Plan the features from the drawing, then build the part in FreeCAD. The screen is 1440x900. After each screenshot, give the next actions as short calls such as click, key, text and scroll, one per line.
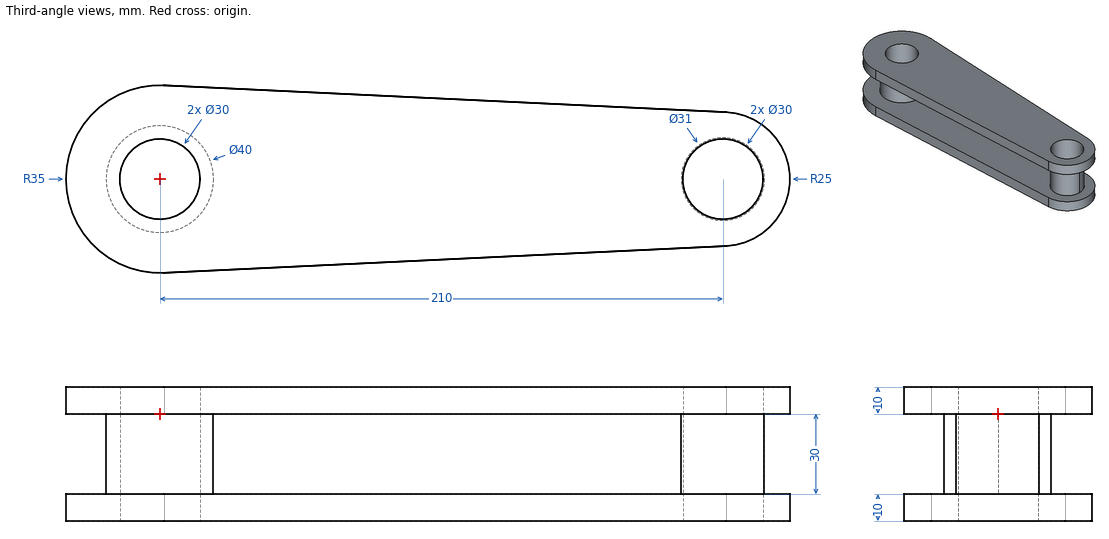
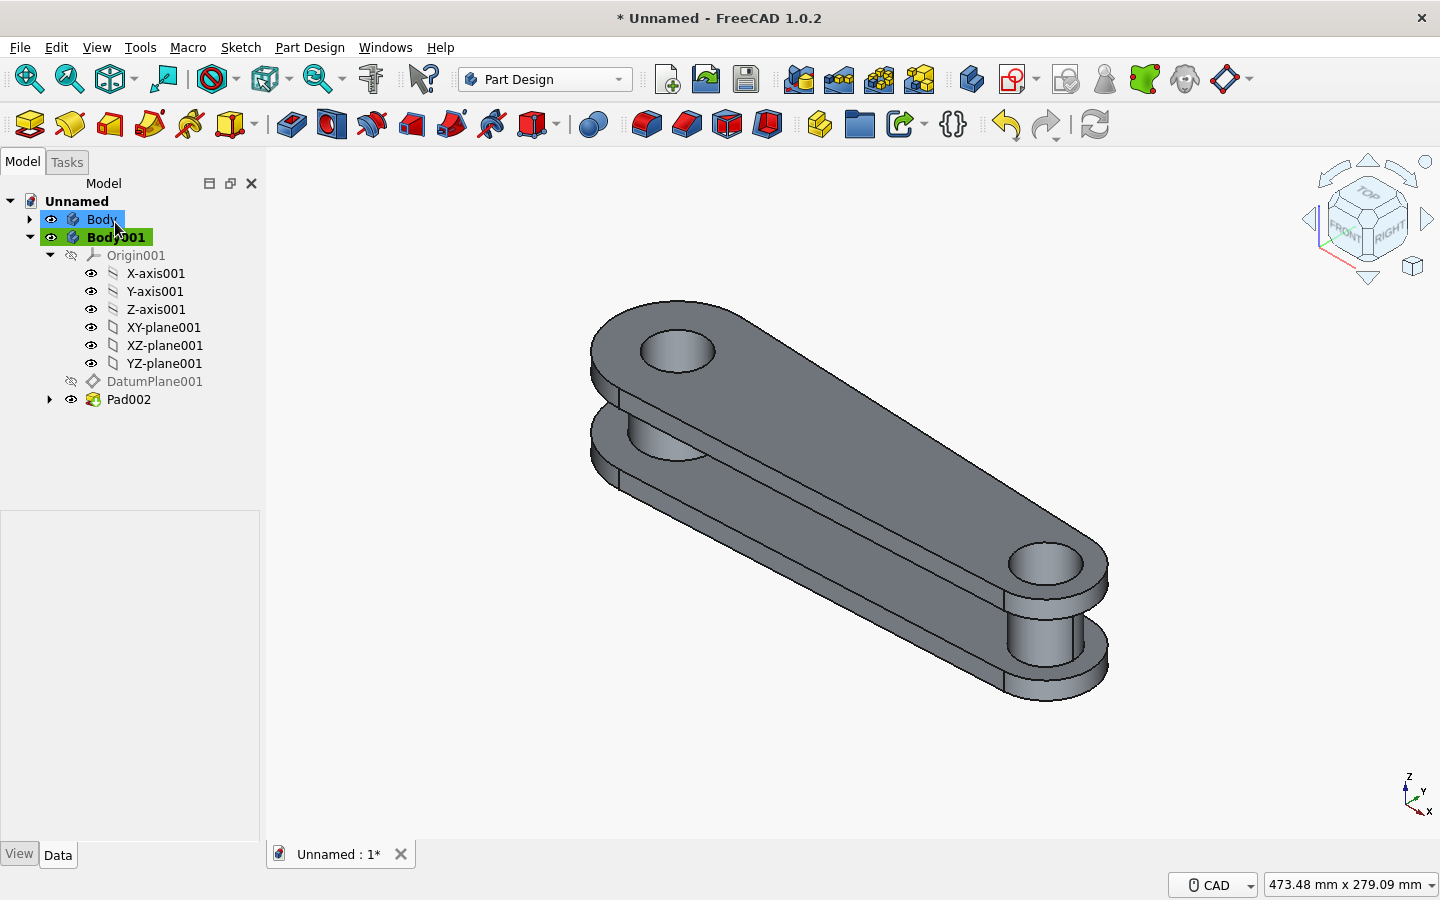
click(700, 465)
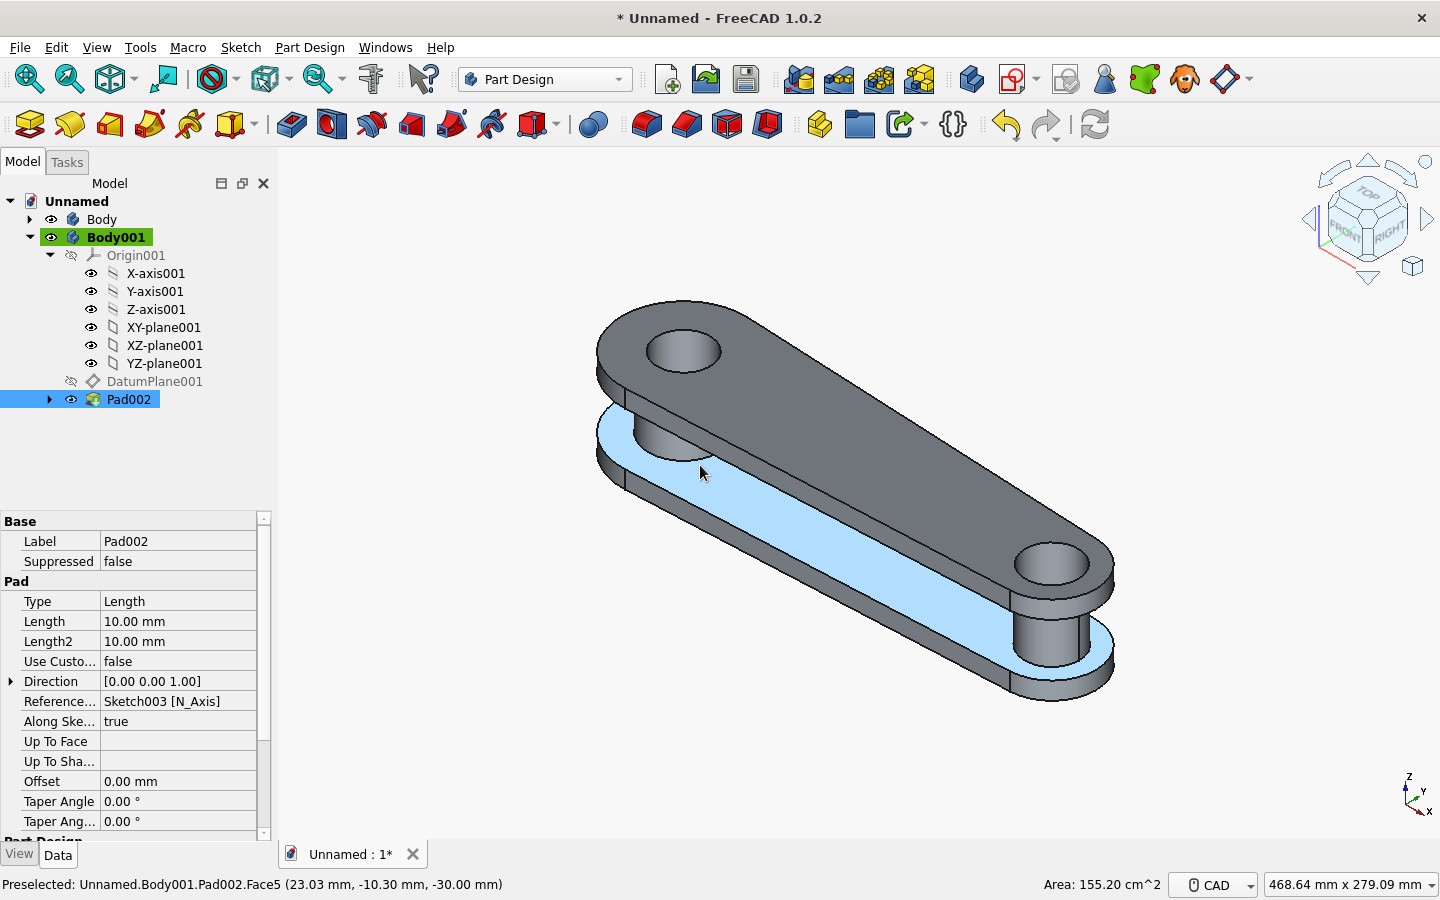
click(1012, 80)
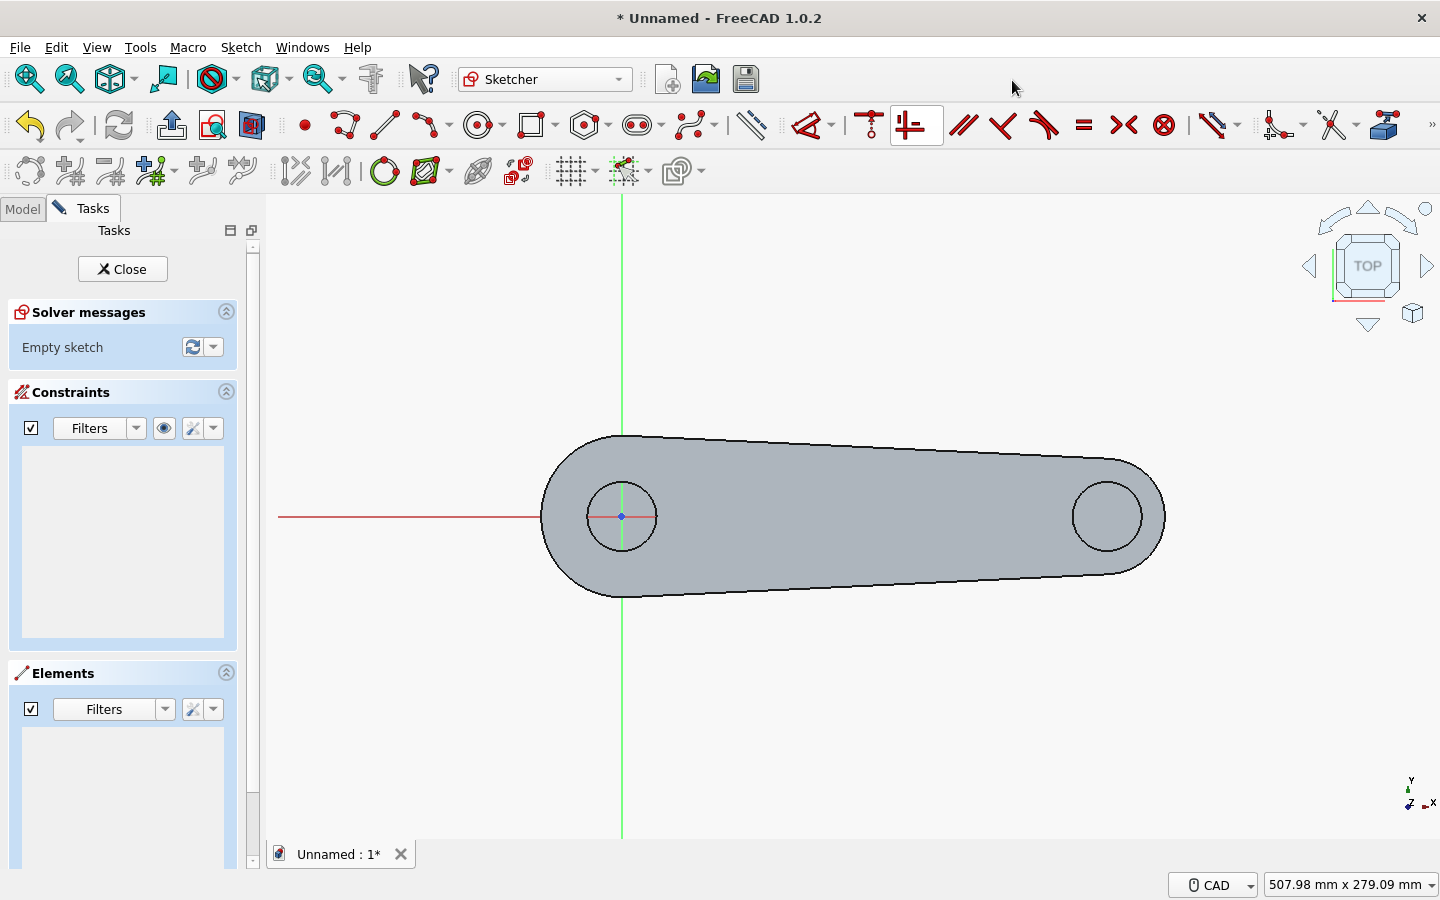
click(478, 126)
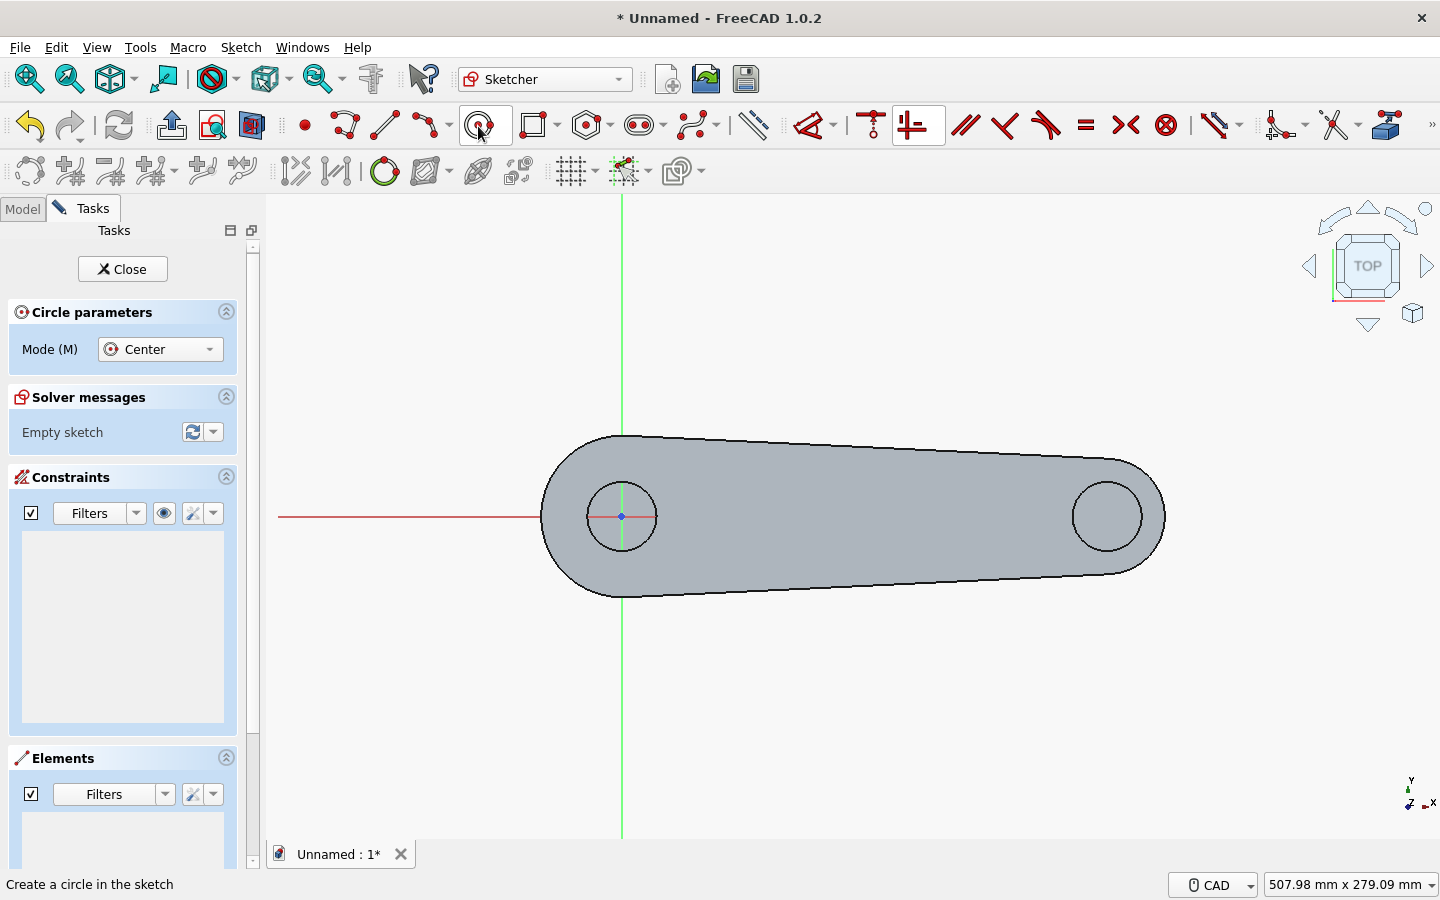
click(1107, 516)
move(1132, 492)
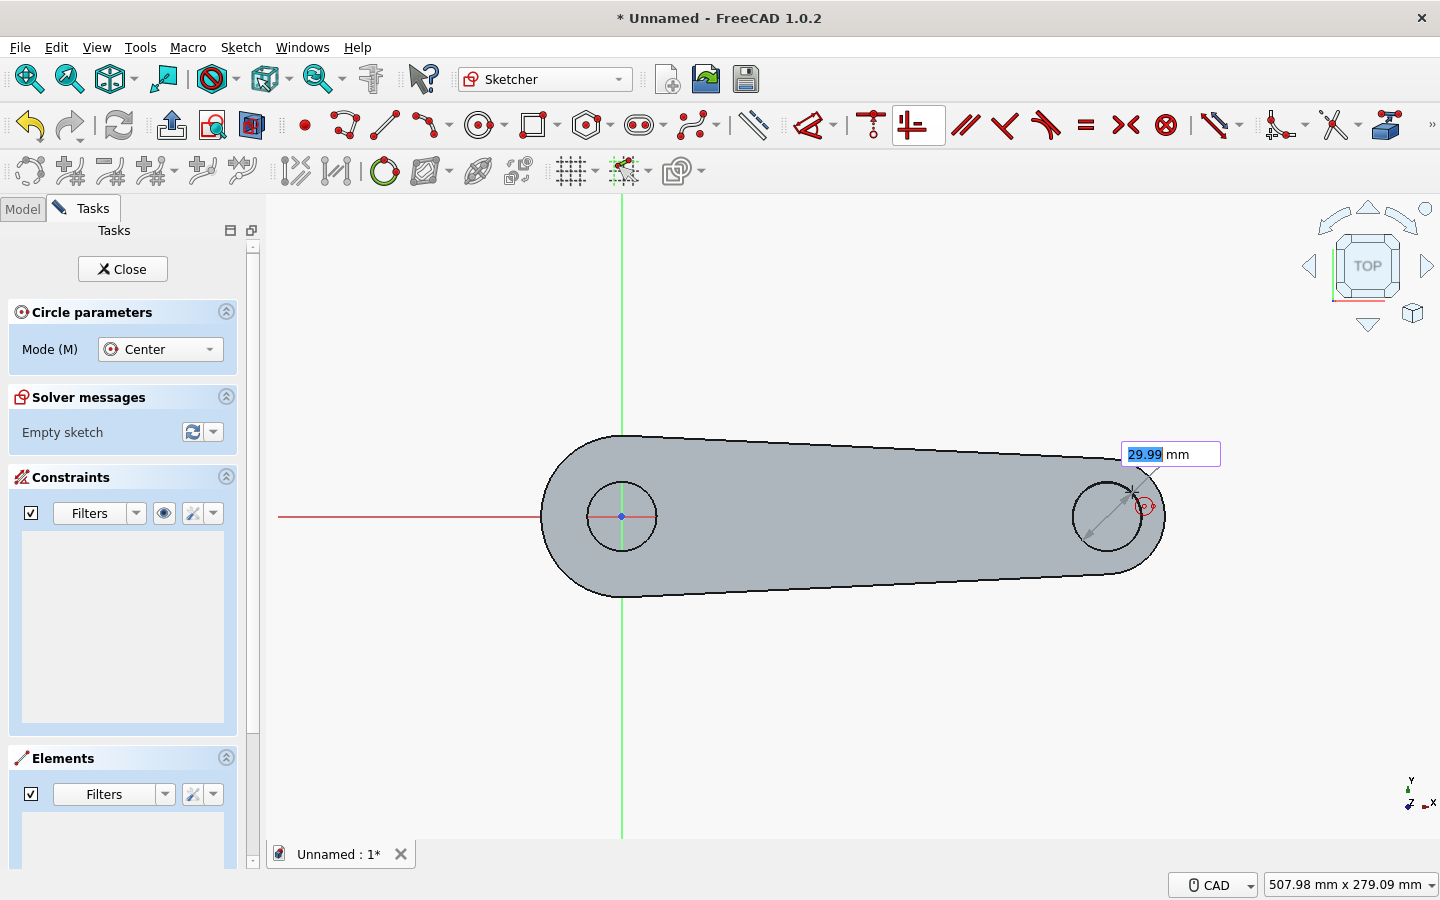
text(30)
key(Return)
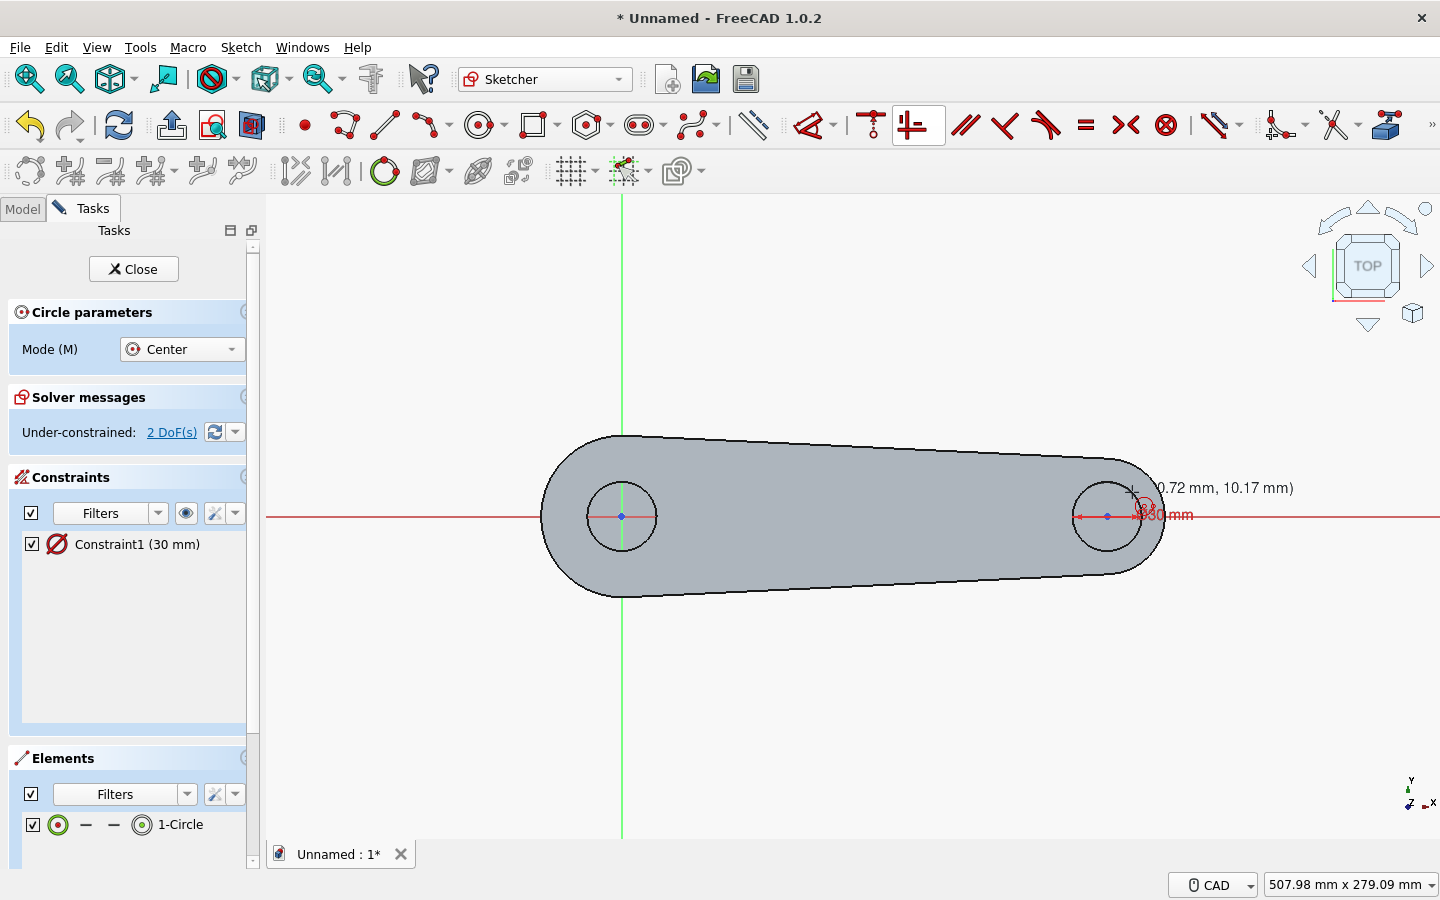
click(622, 516)
move(646, 492)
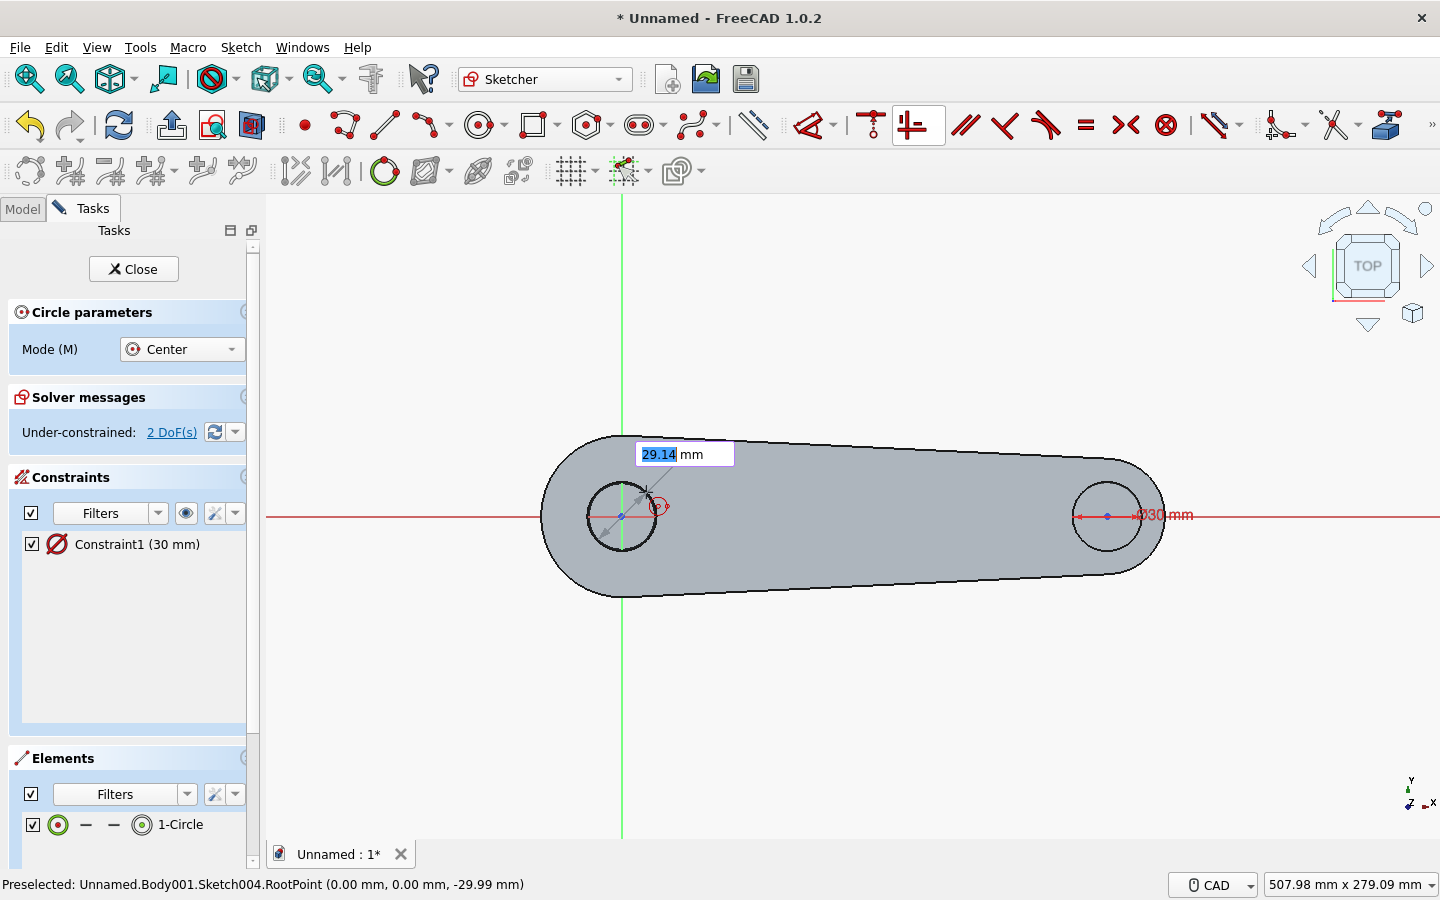
text(30)
key(Return)
key(Escape)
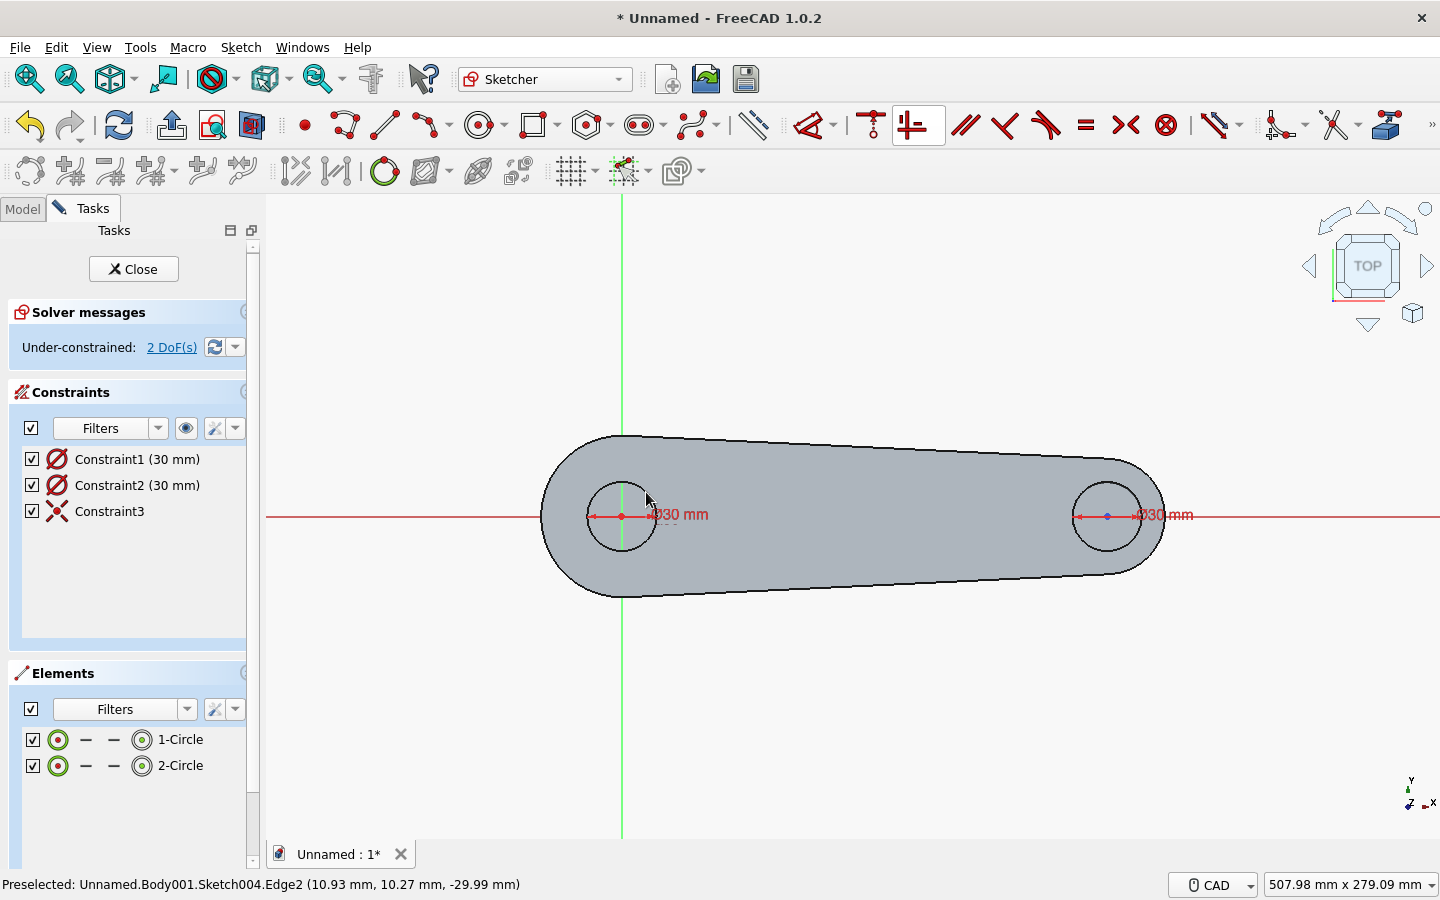
click(1107, 517)